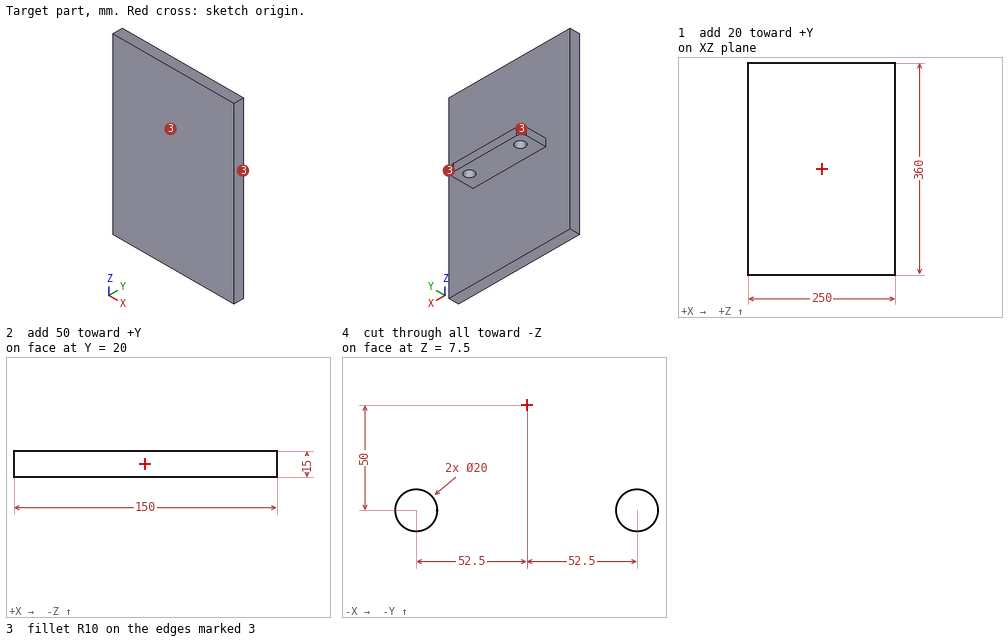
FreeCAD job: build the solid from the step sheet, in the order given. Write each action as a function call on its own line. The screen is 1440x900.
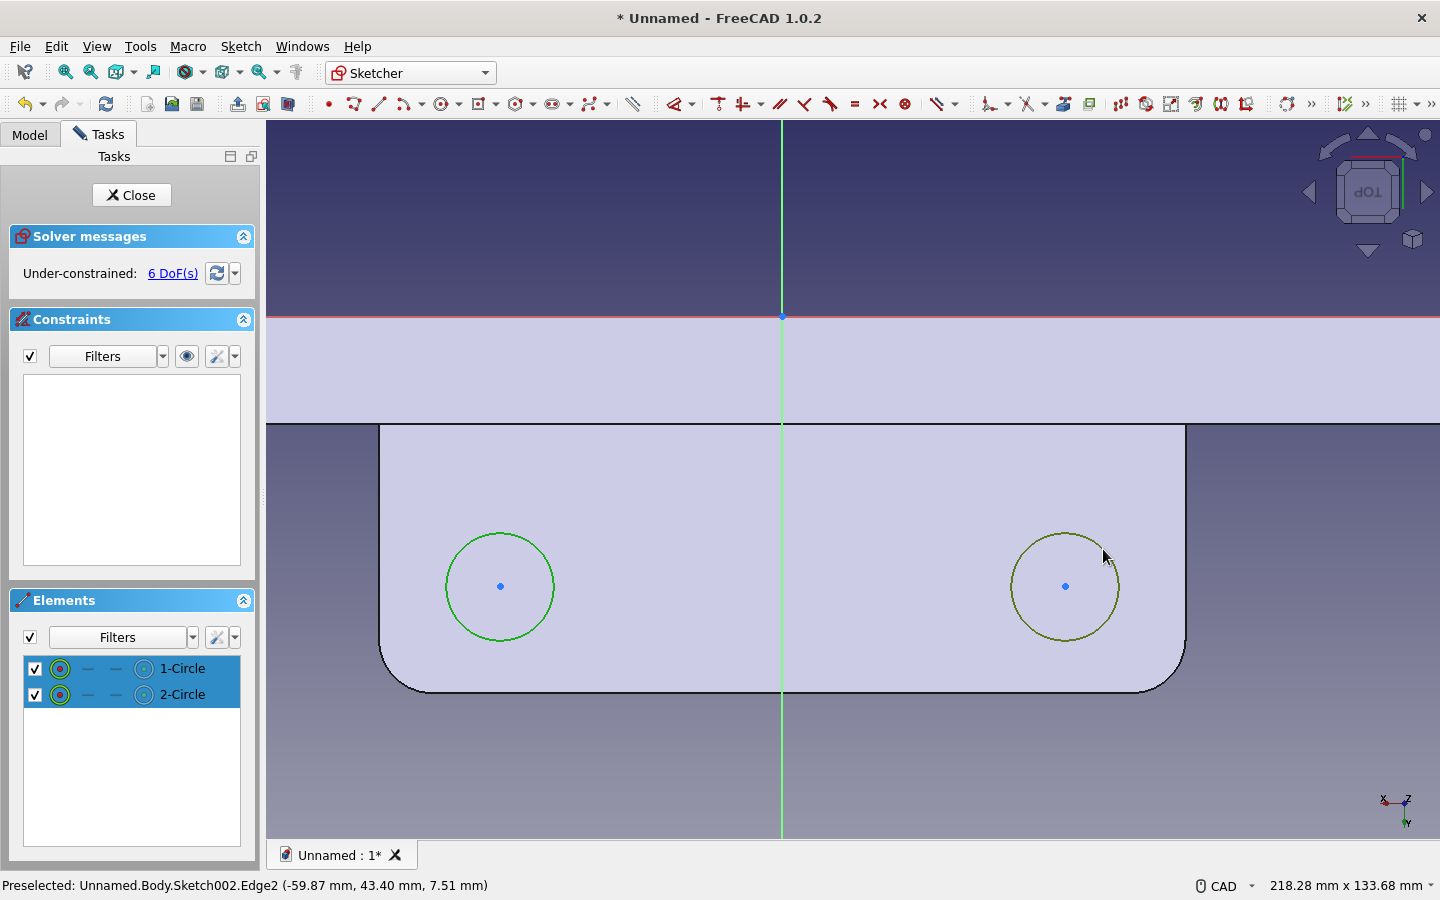
key(e)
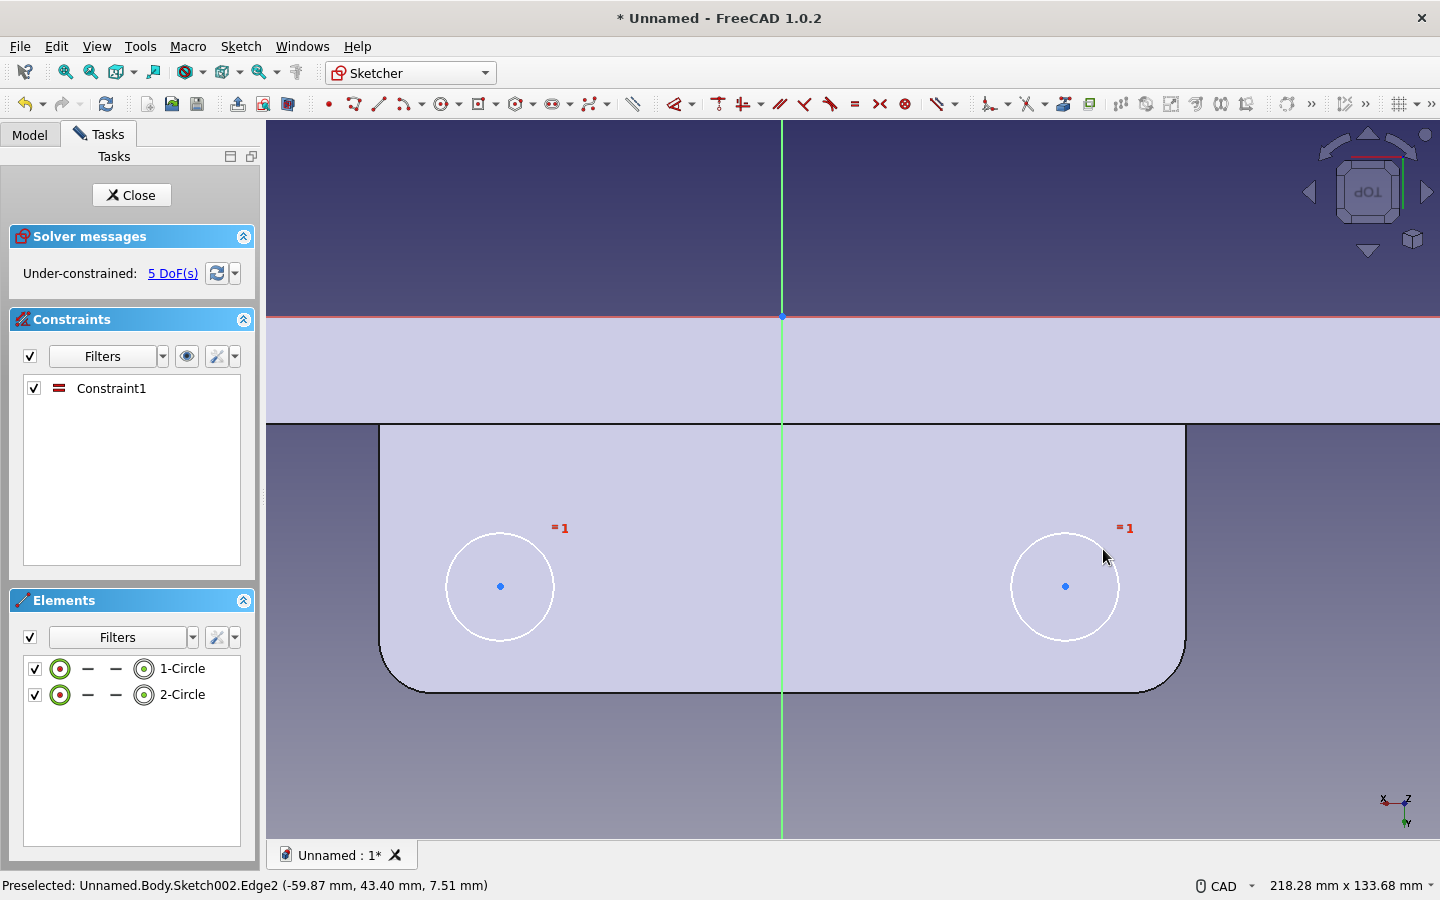
click(500, 587)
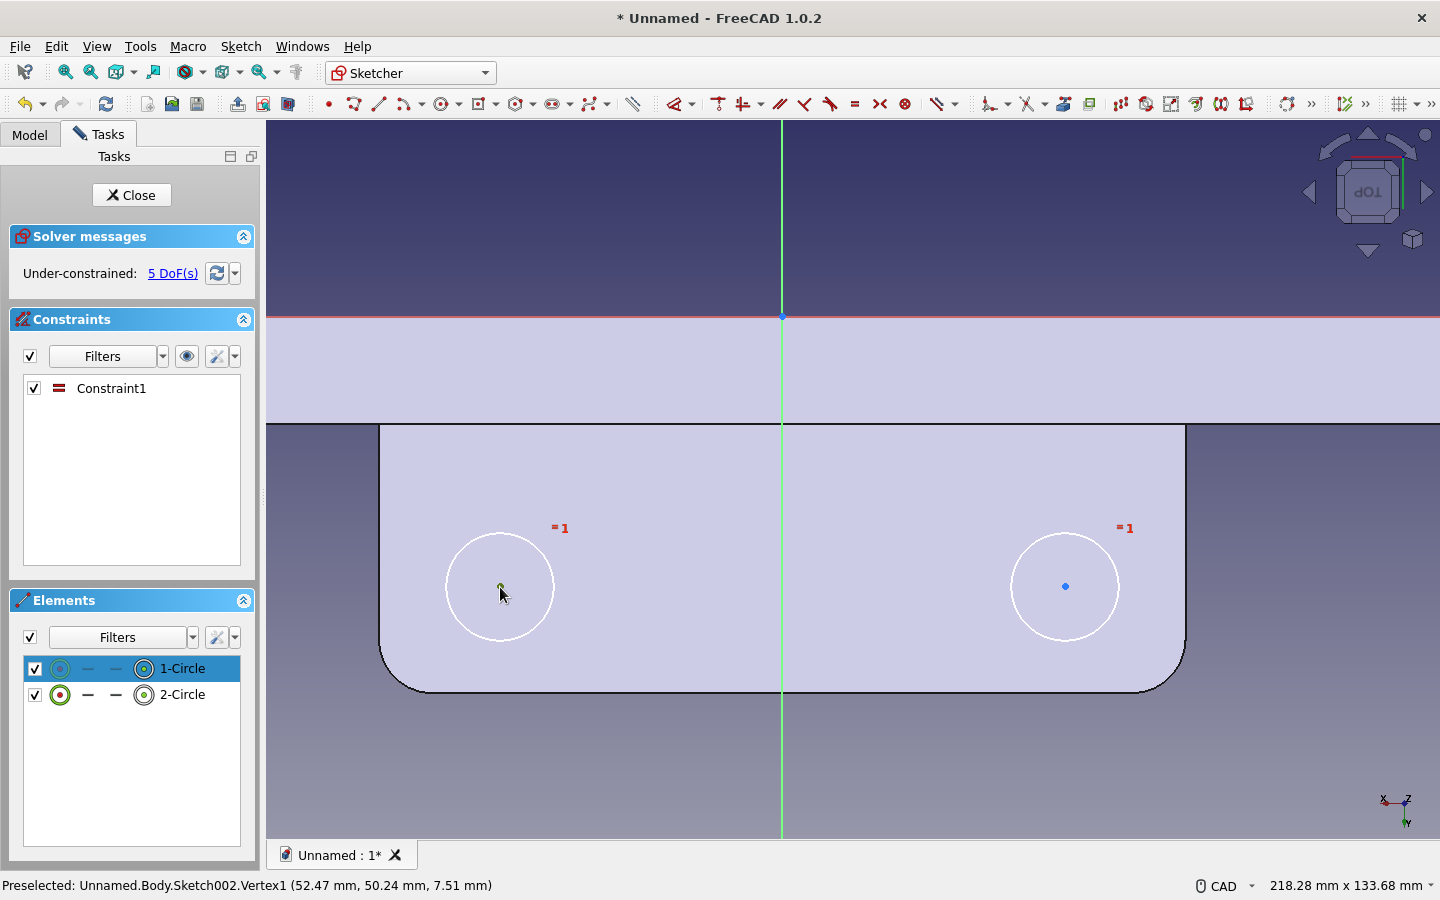
click(1065, 587)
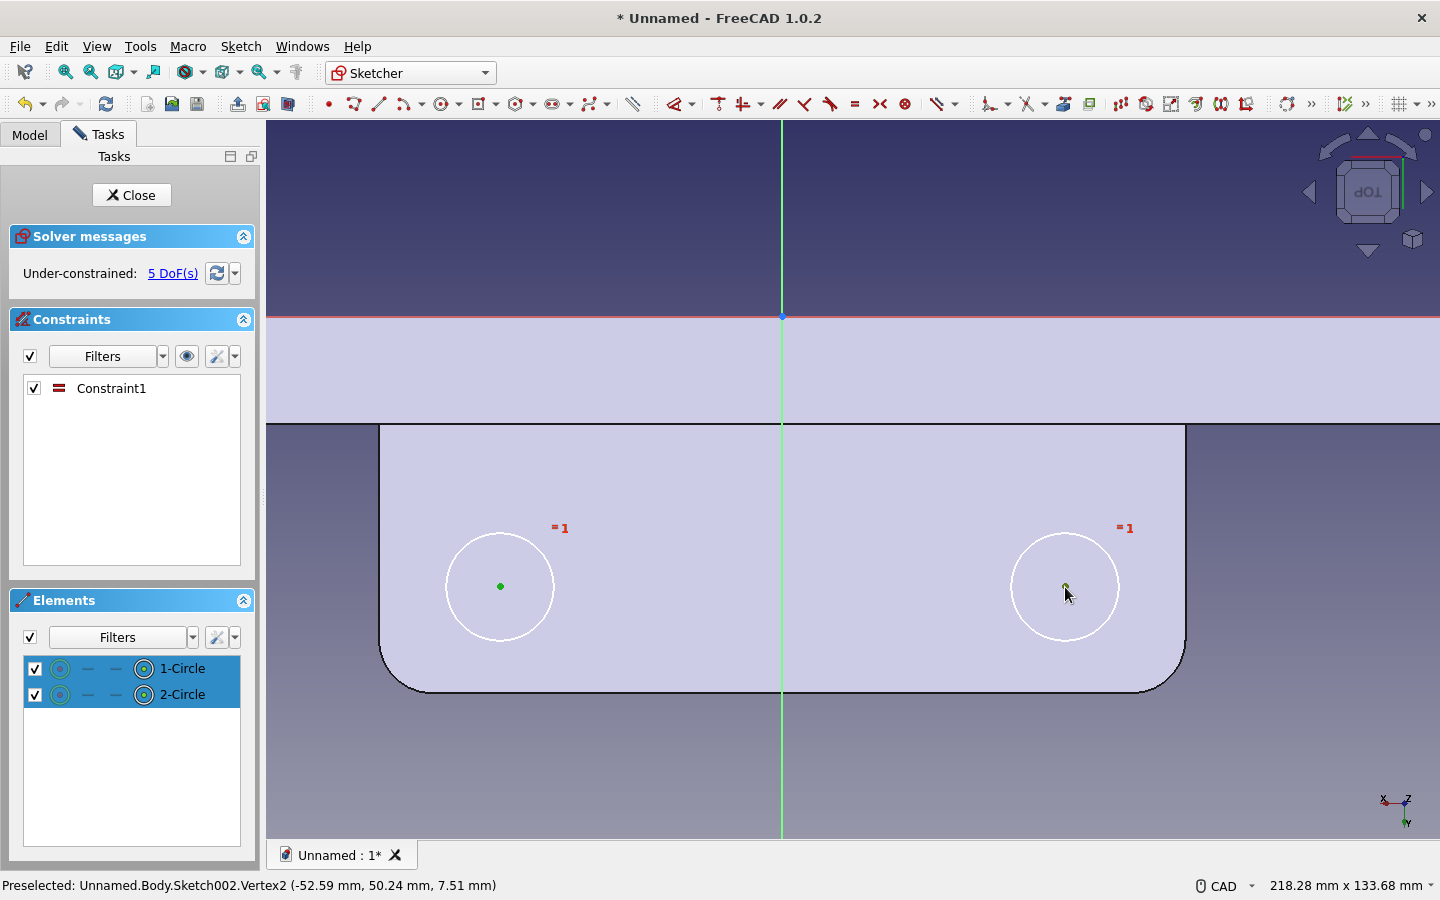
key(h)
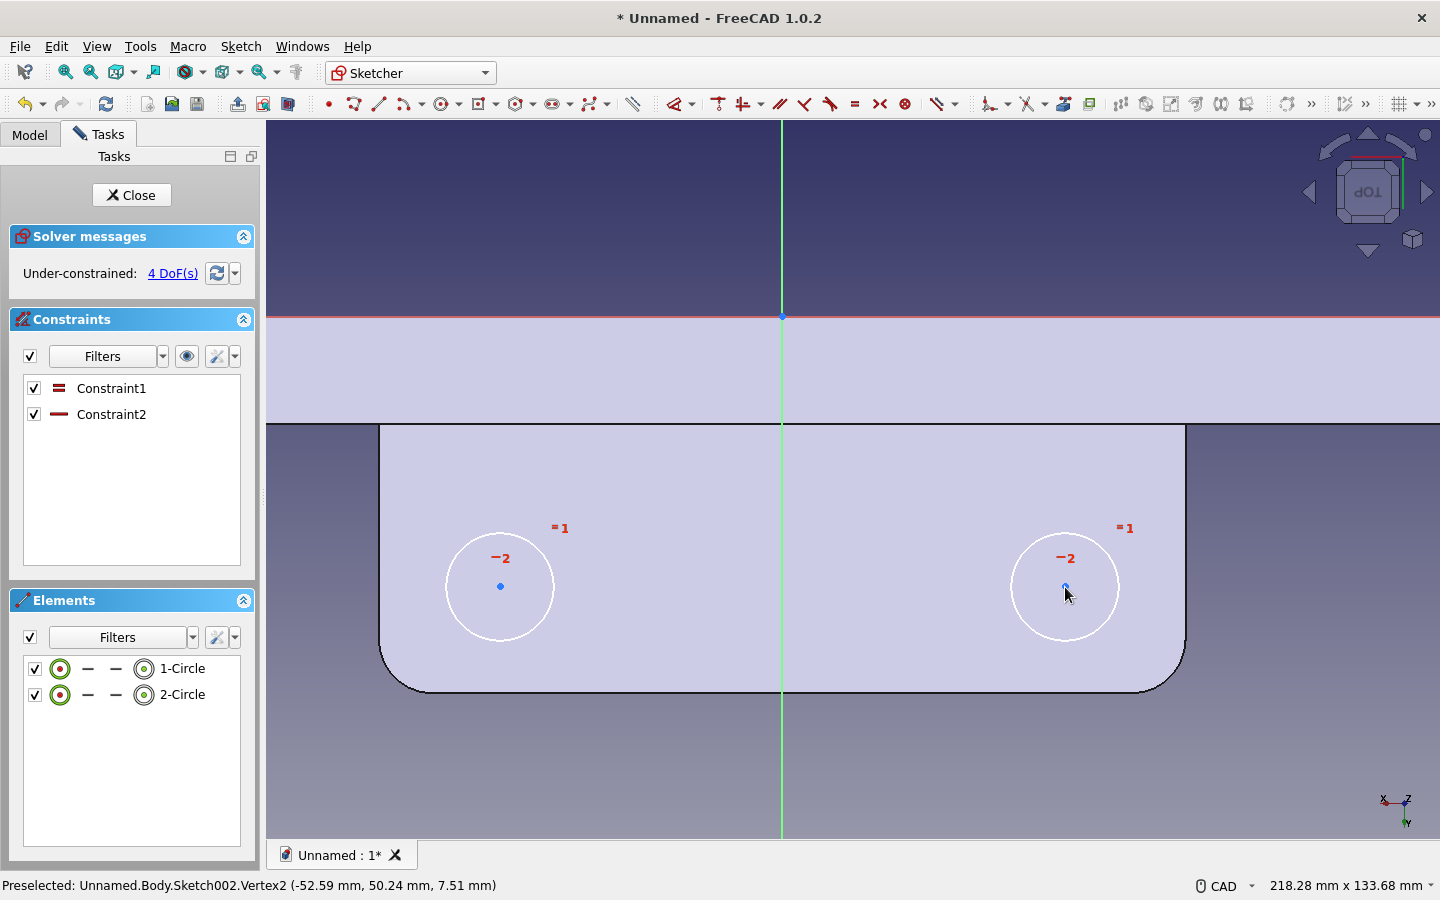
key(d)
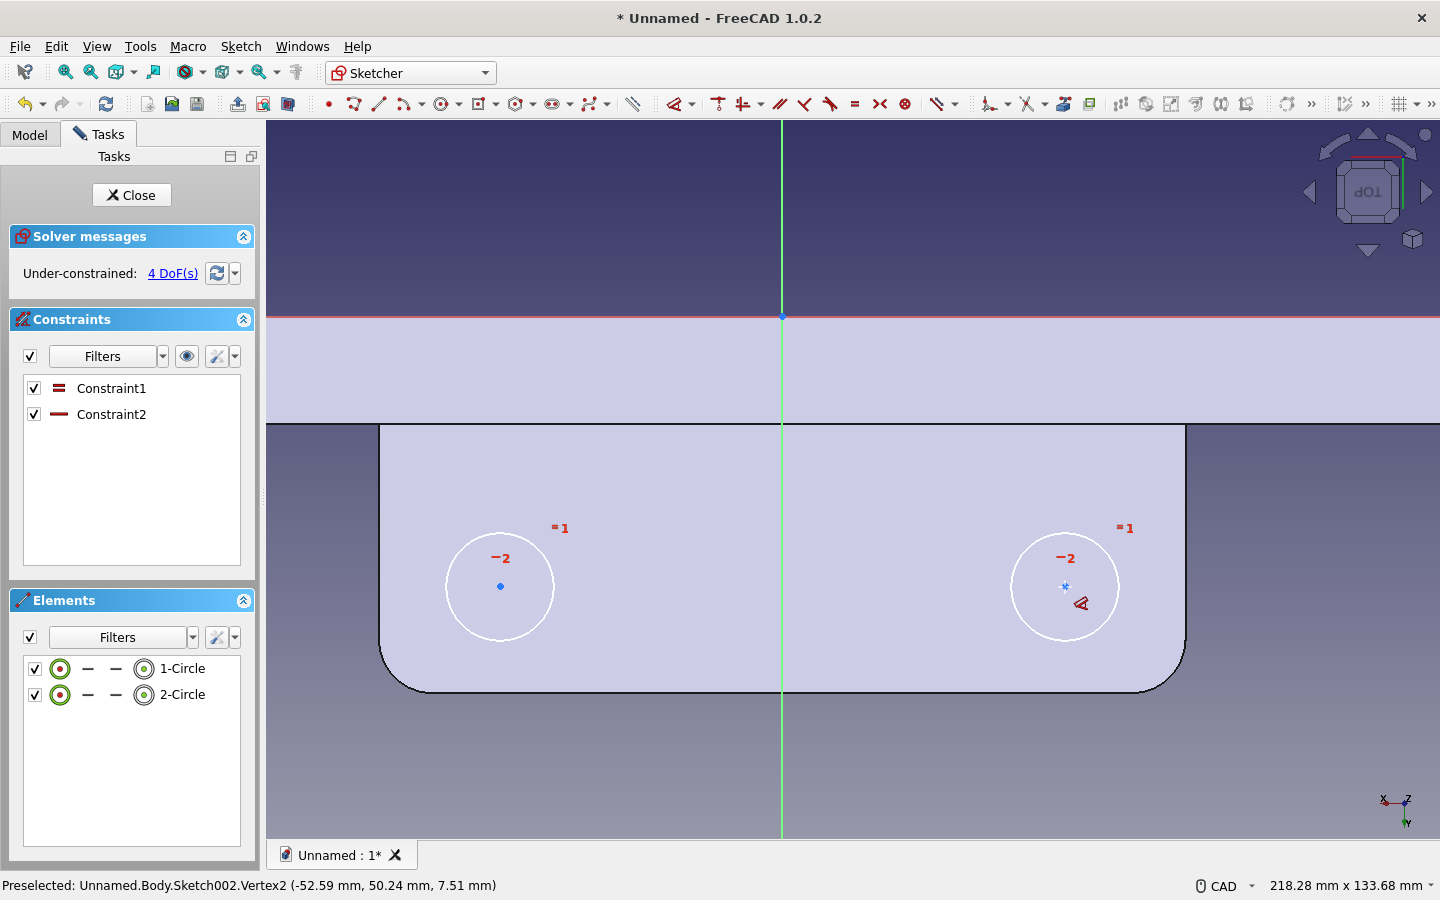
click(538, 549)
click(561, 526)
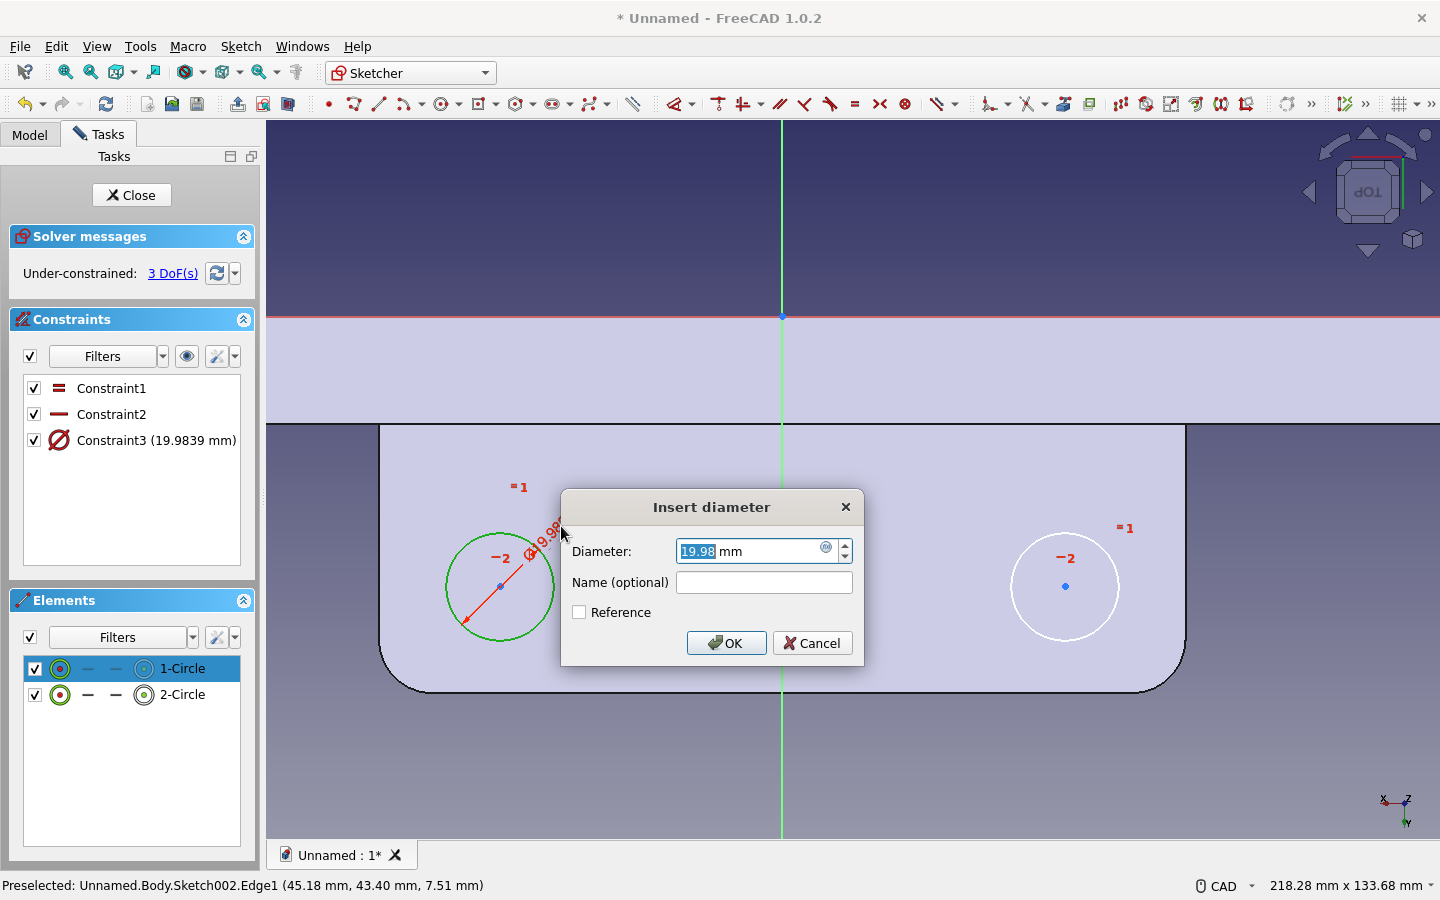
text(20)
key(Return)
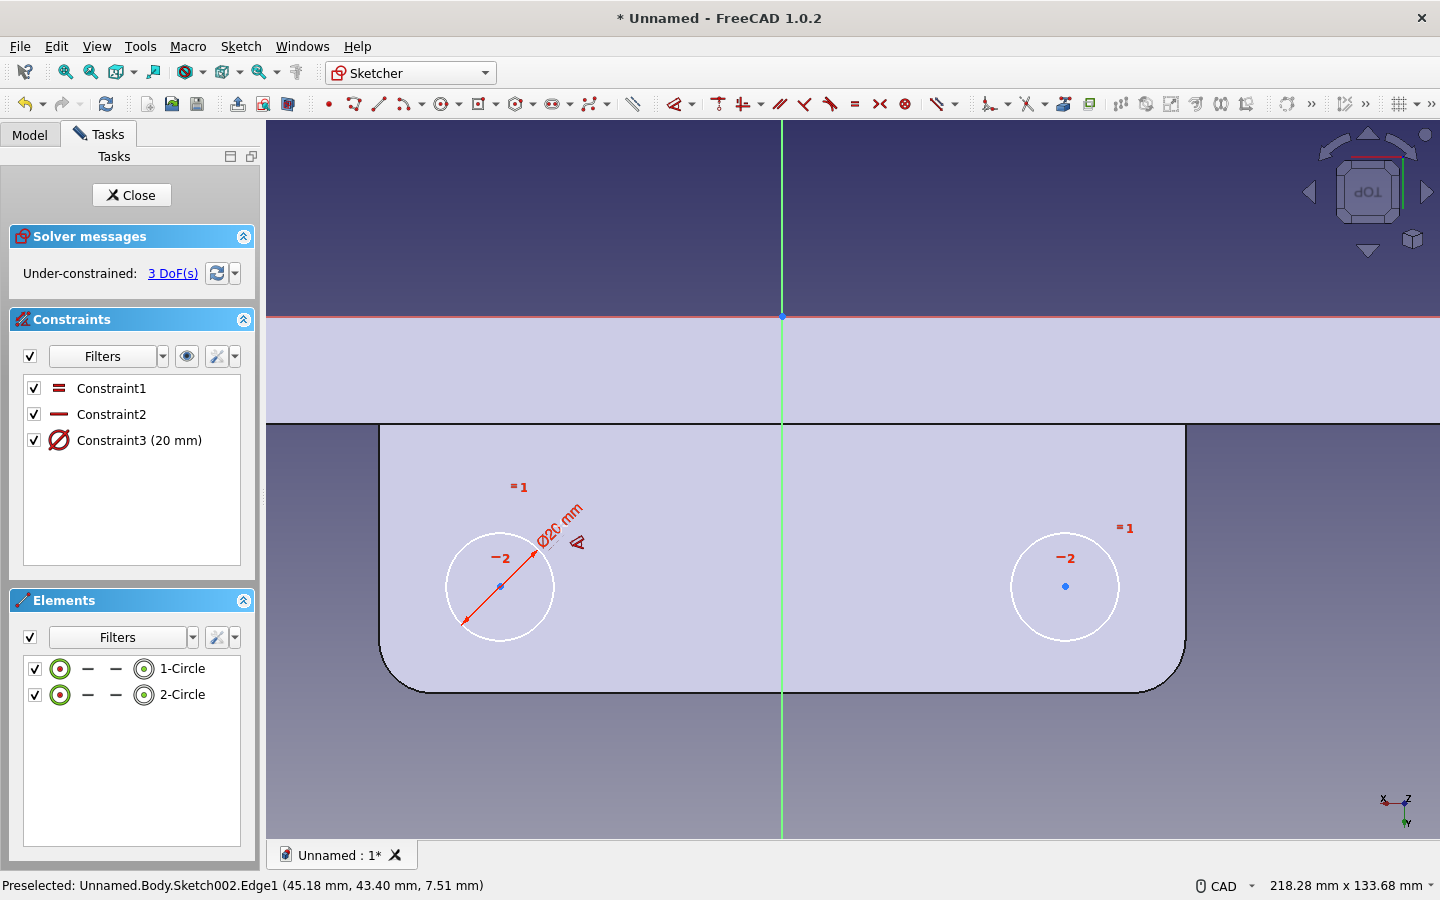
click(500, 587)
click(466, 452)